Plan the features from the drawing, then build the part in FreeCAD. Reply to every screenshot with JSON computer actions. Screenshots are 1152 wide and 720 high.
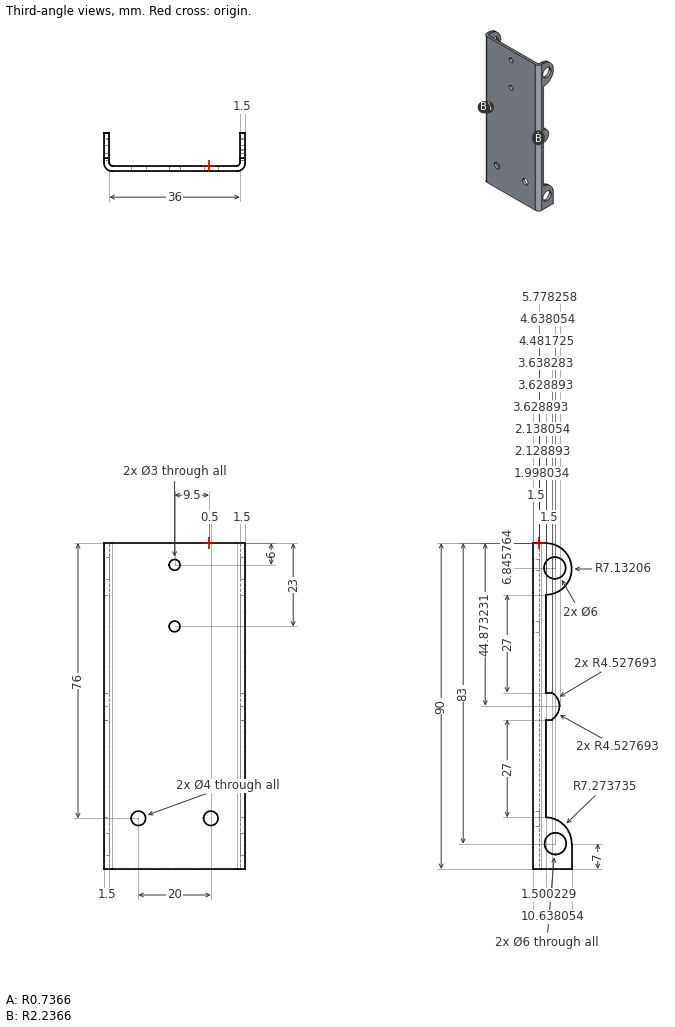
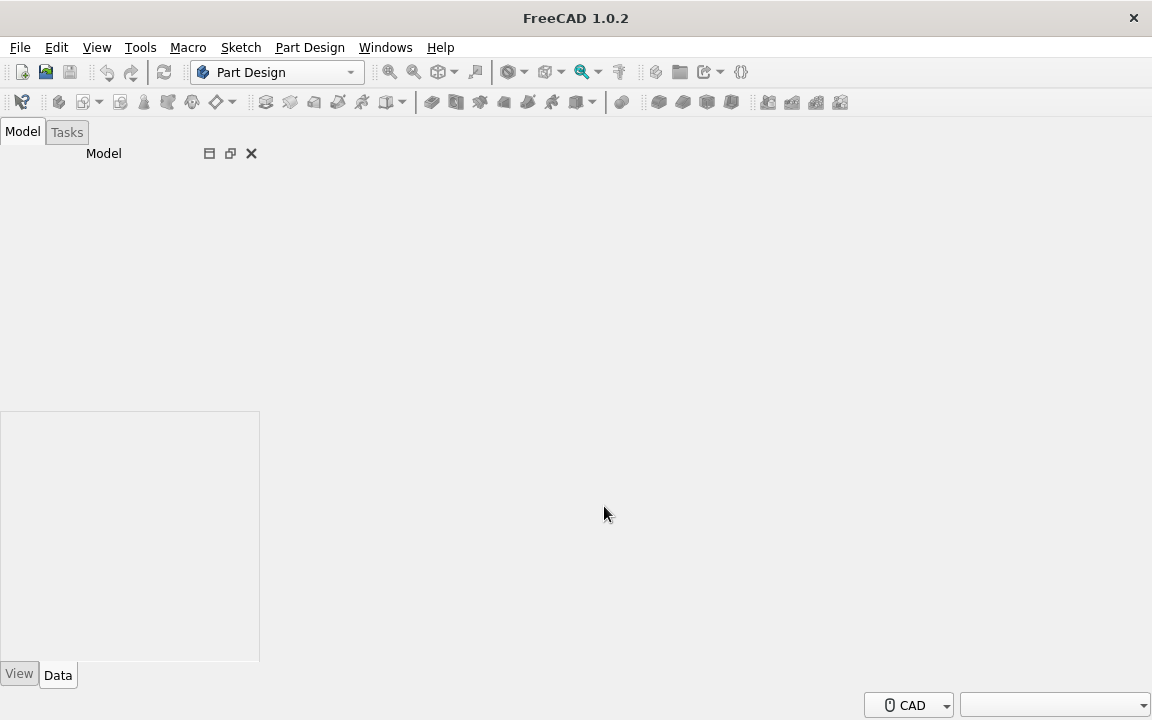
{"action": "key", "text": "ctrl+n"}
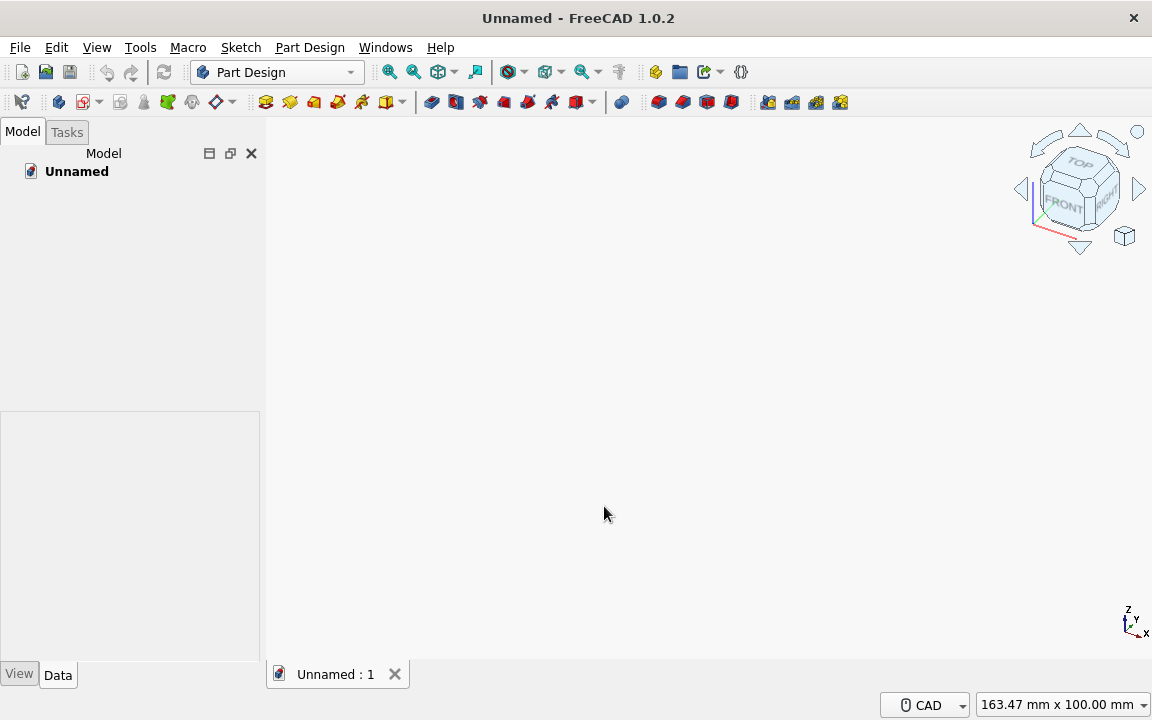
{"action": "left_click", "coordinate": [60, 102]}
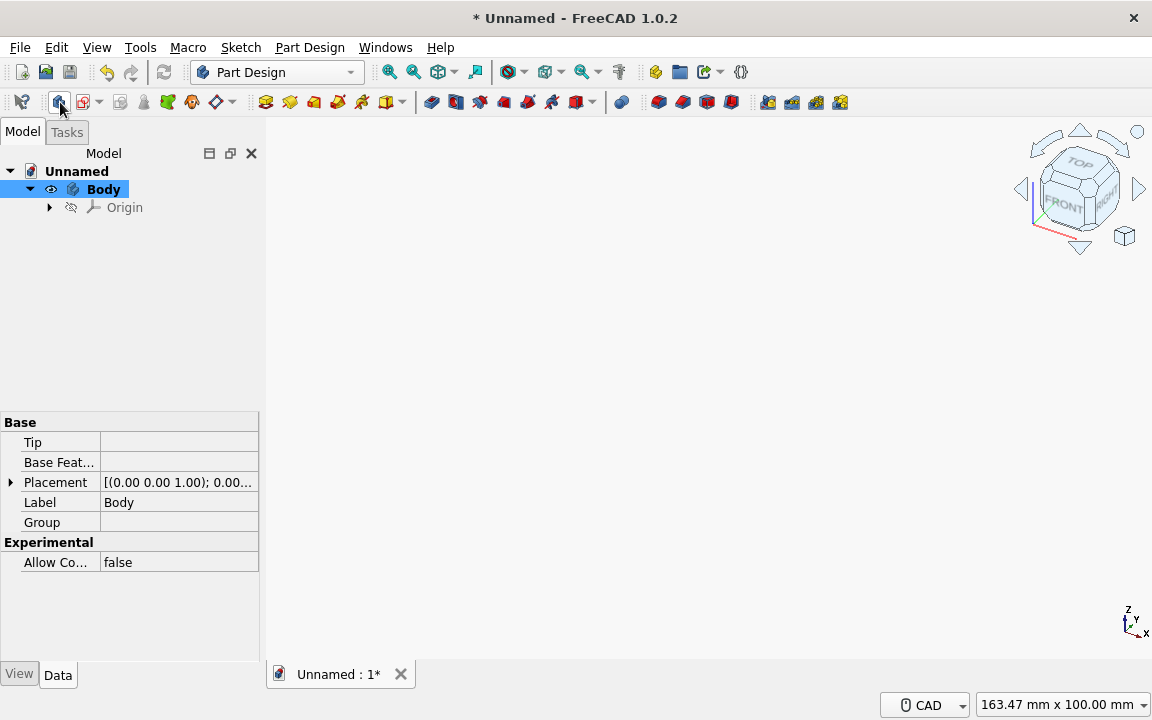
{"action": "left_click", "coordinate": [50, 207]}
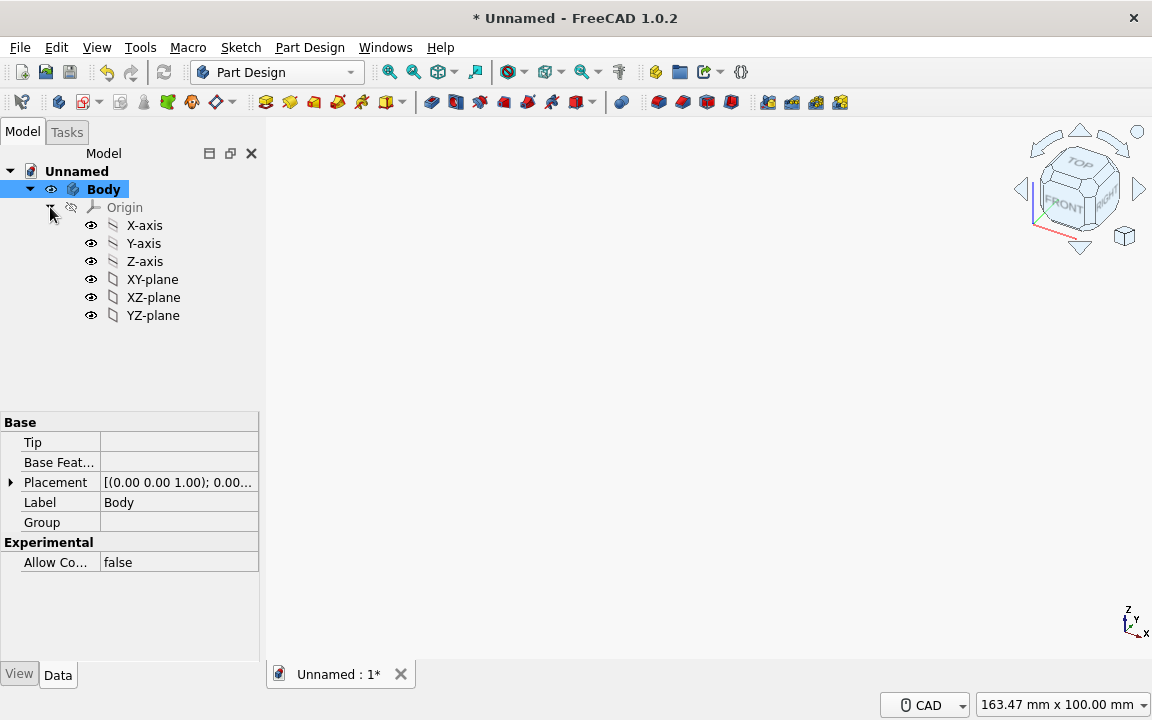
{"action": "left_click", "coordinate": [136, 315]}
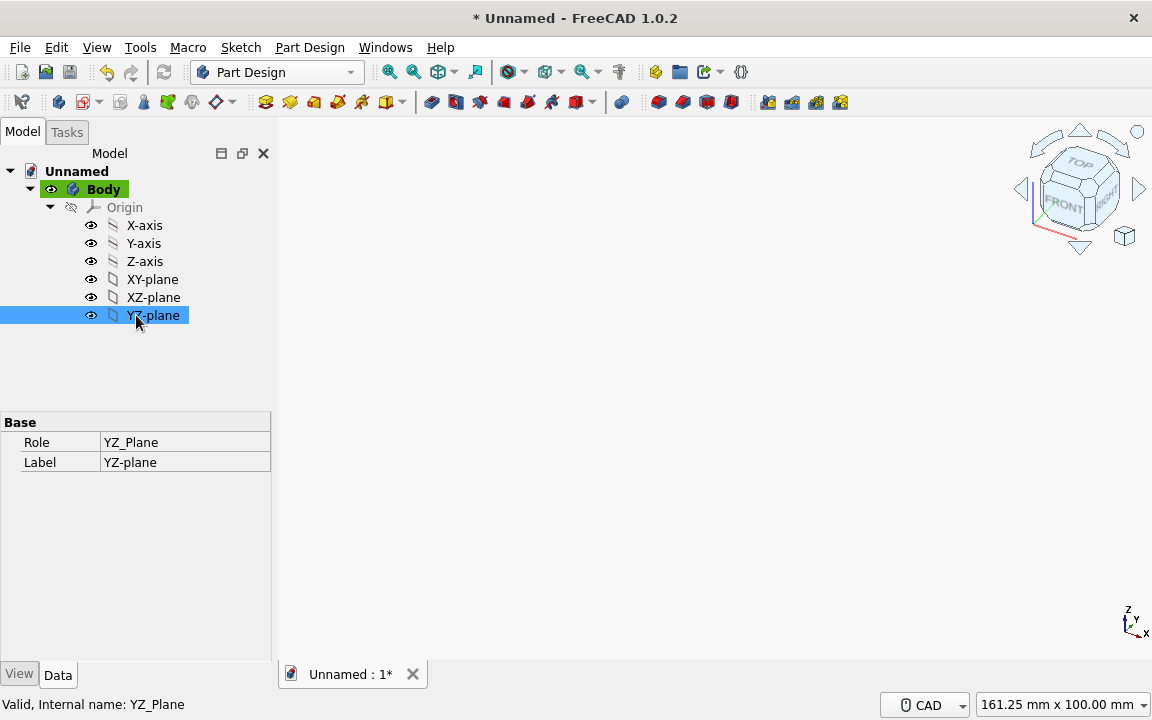
{"action": "left_click", "coordinate": [216, 102]}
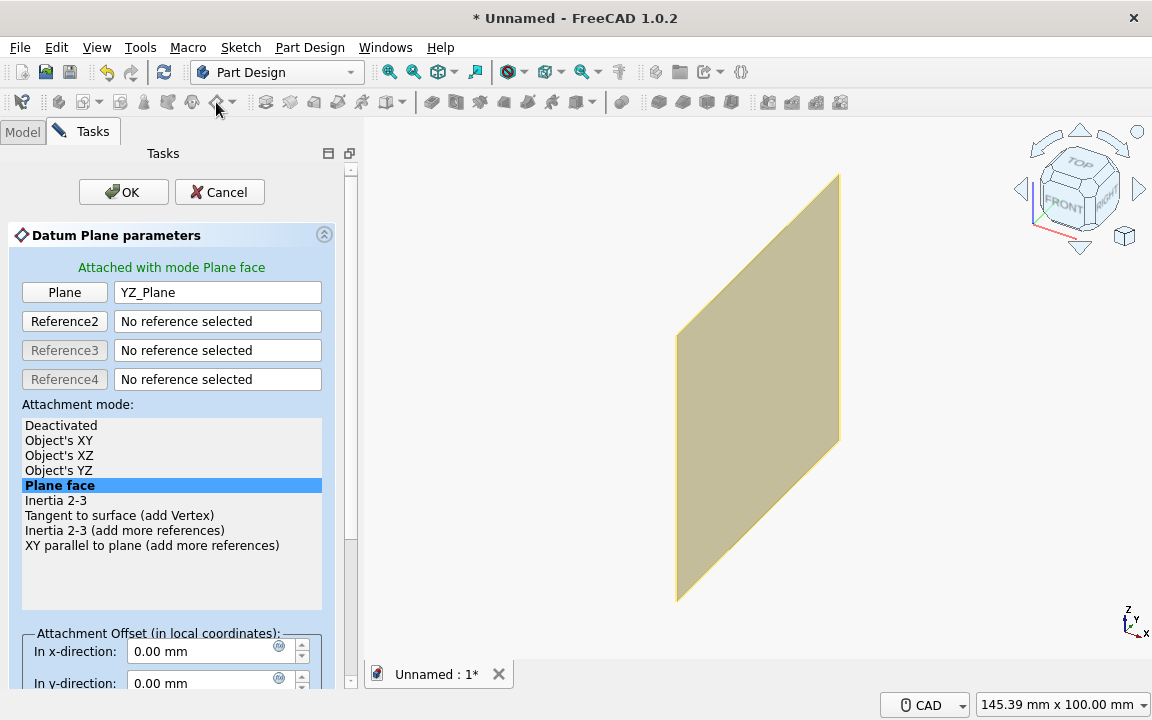
{"action": "scroll", "coordinate": [351, 426], "scroll_direction": "down", "scroll_amount": 2}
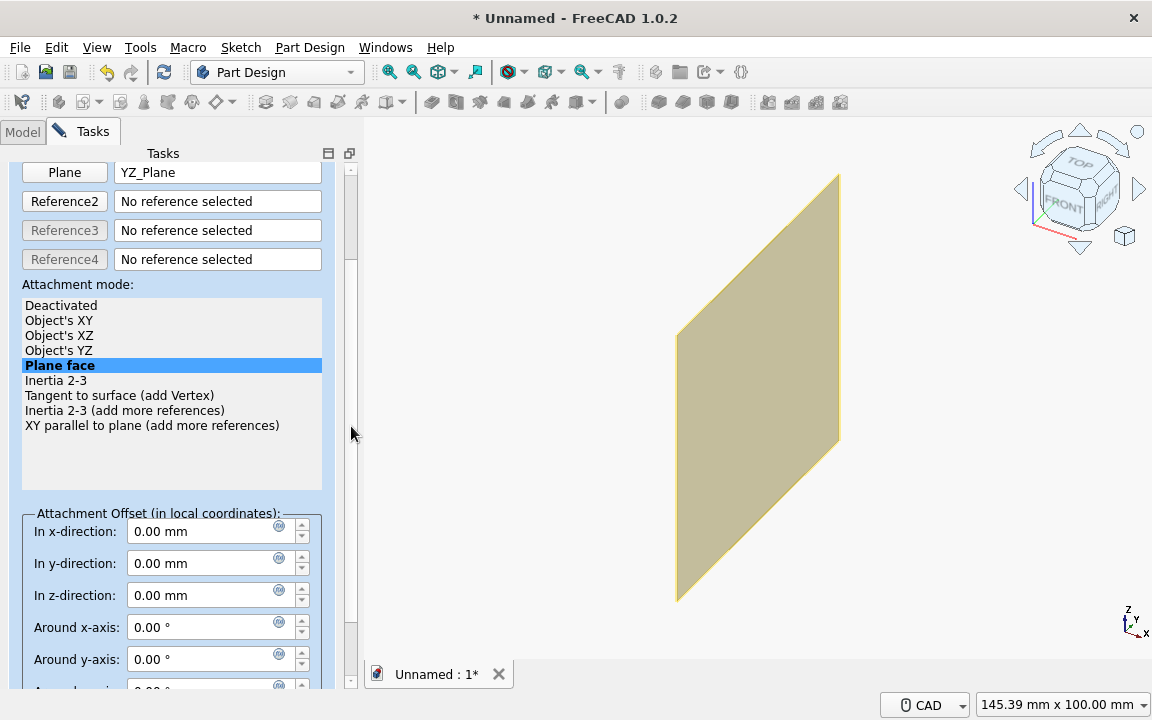
{"action": "triple_click", "coordinate": [210, 595]}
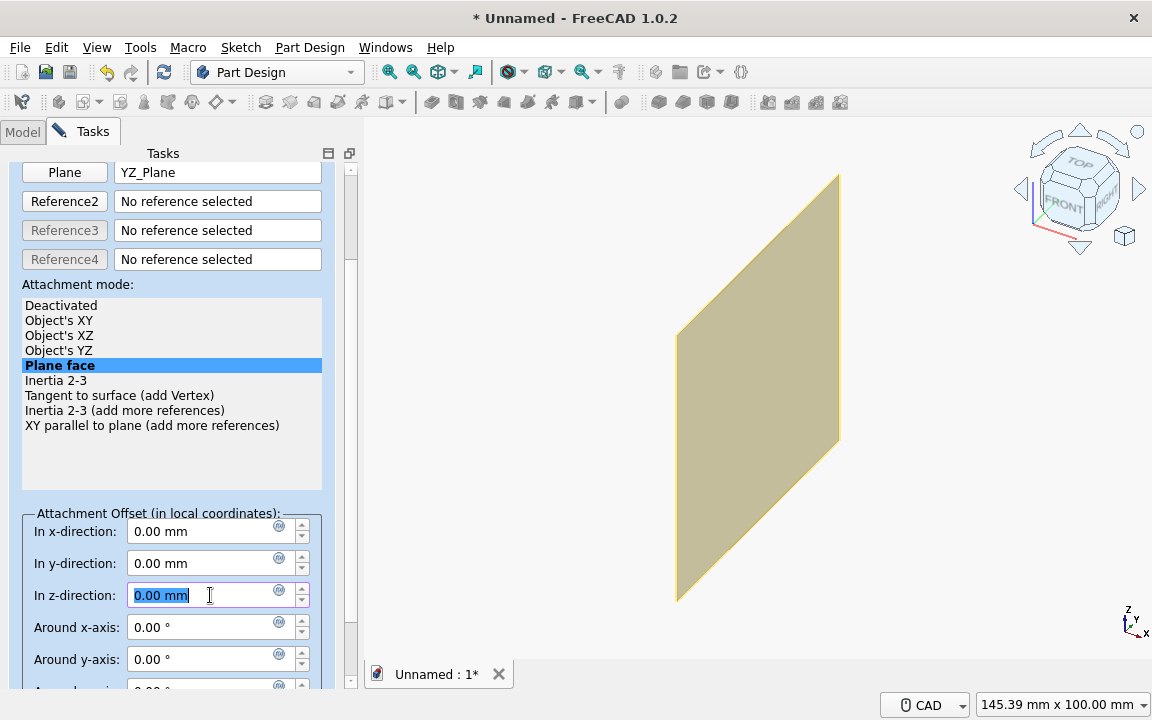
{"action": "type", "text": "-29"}
{"action": "key", "text": "Tab"}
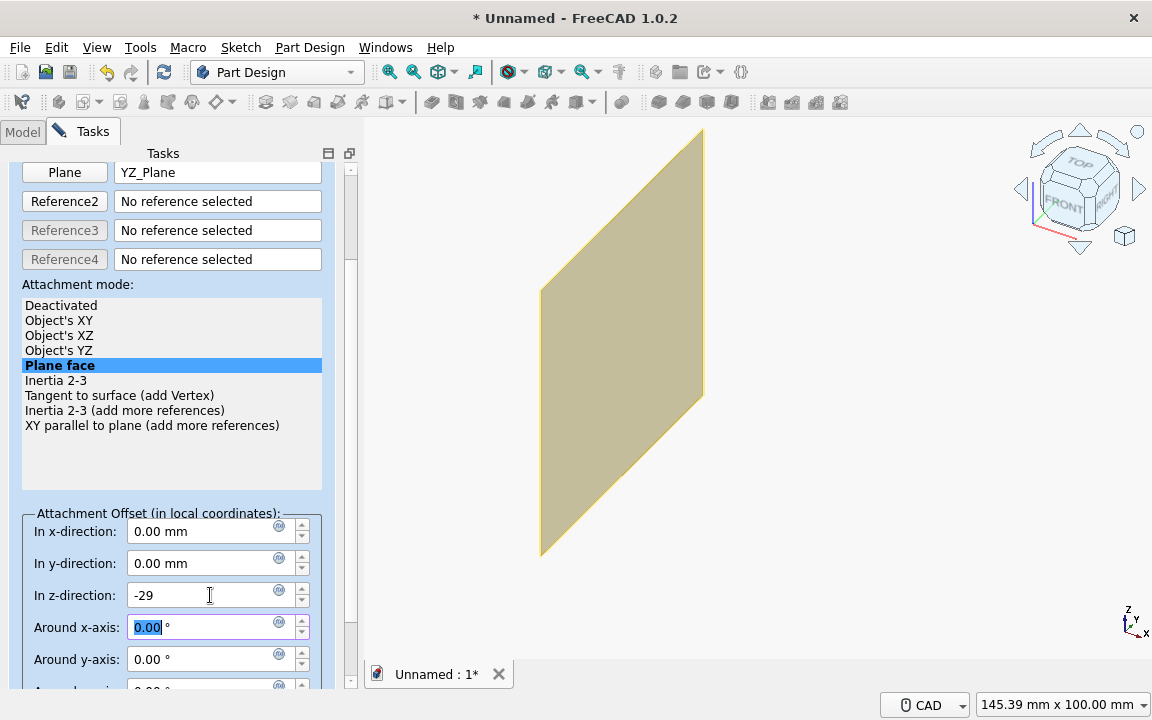
{"action": "scroll", "coordinate": [351, 426], "scroll_direction": "up", "scroll_amount": 3}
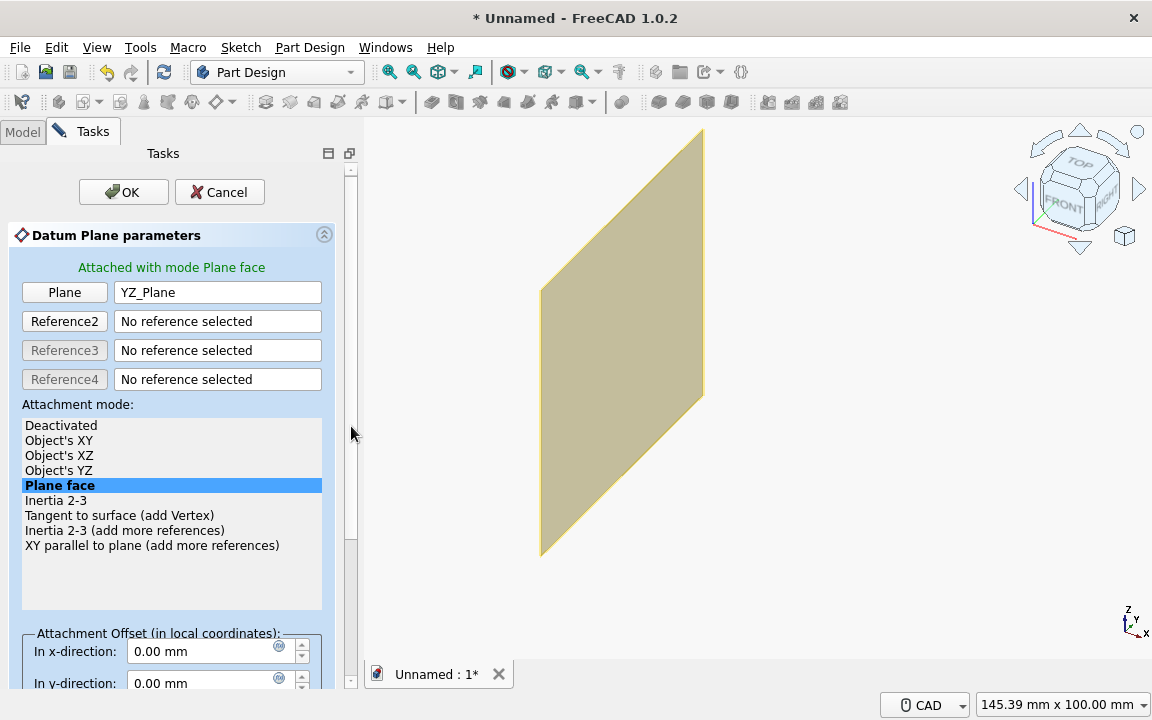
{"action": "left_click", "coordinate": [124, 192]}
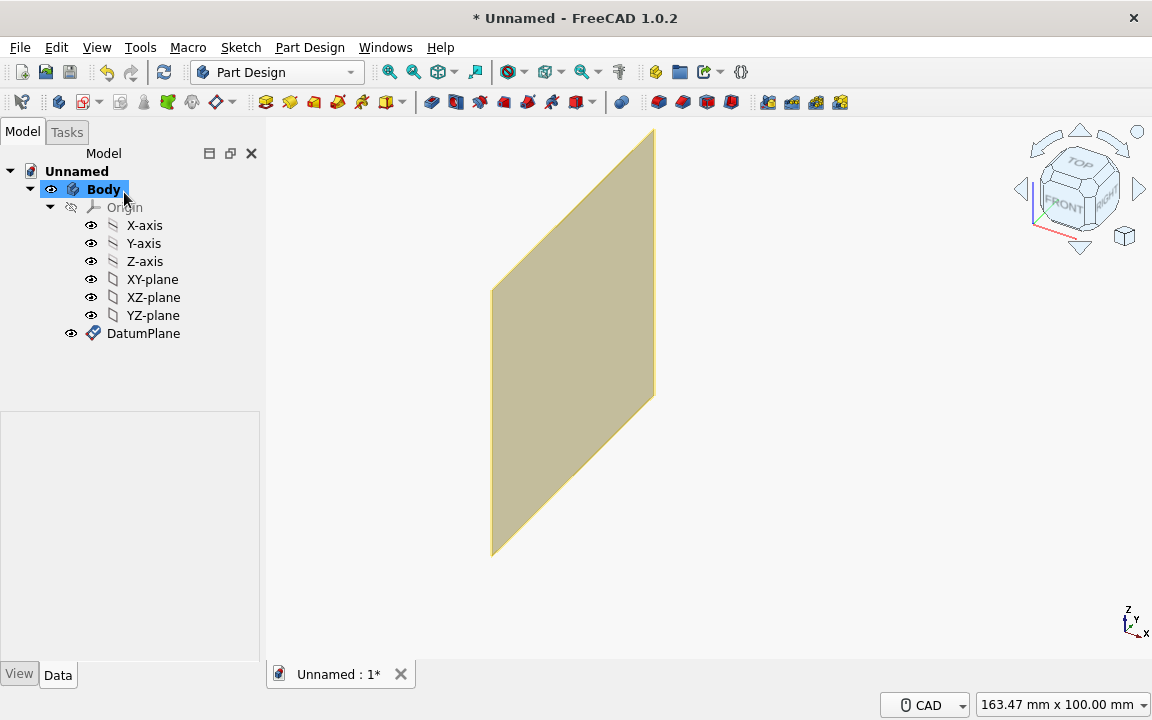
{"action": "left_click", "coordinate": [116, 333]}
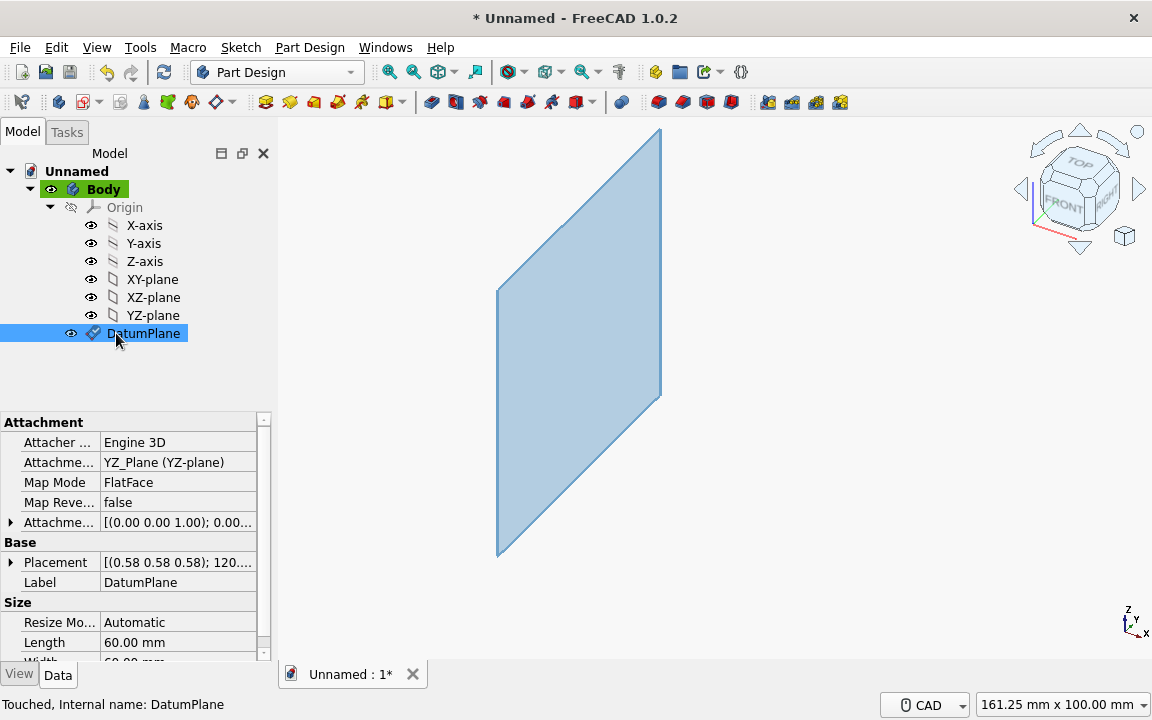
{"action": "left_click", "coordinate": [84, 102]}